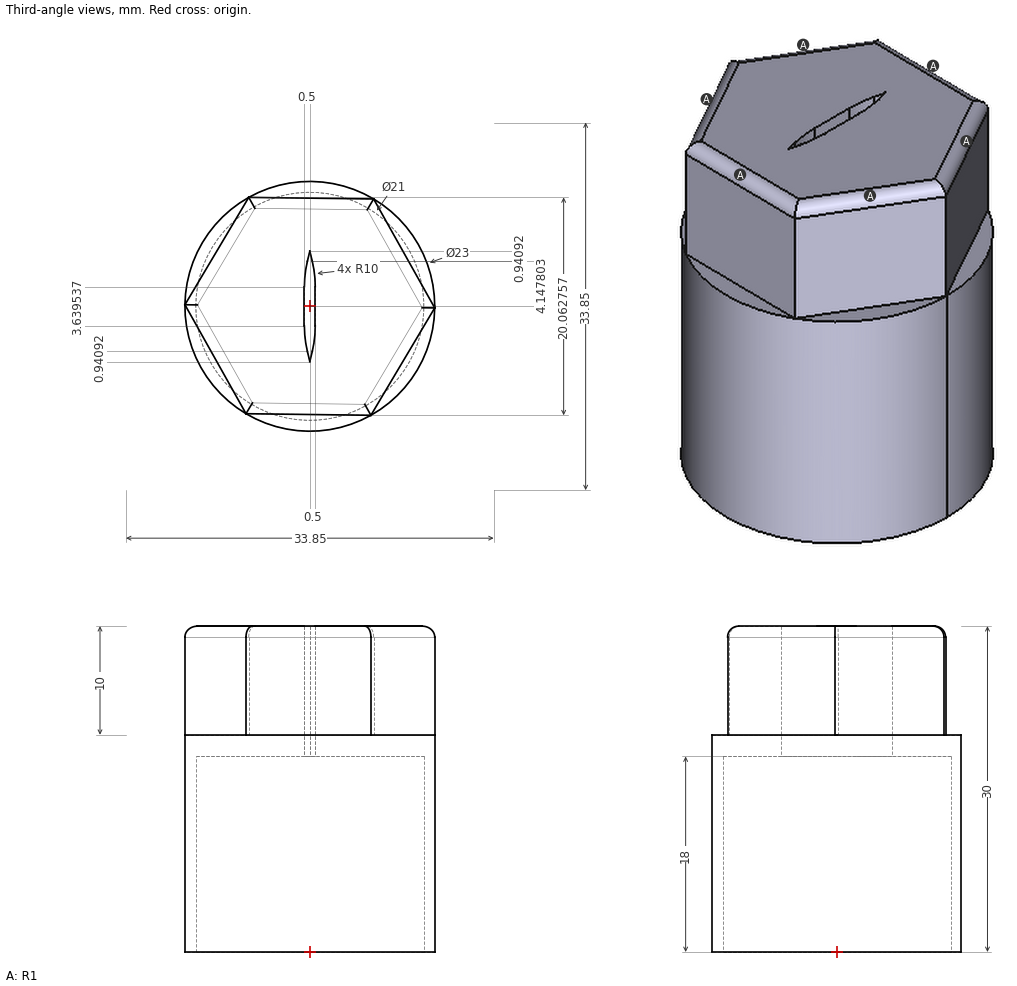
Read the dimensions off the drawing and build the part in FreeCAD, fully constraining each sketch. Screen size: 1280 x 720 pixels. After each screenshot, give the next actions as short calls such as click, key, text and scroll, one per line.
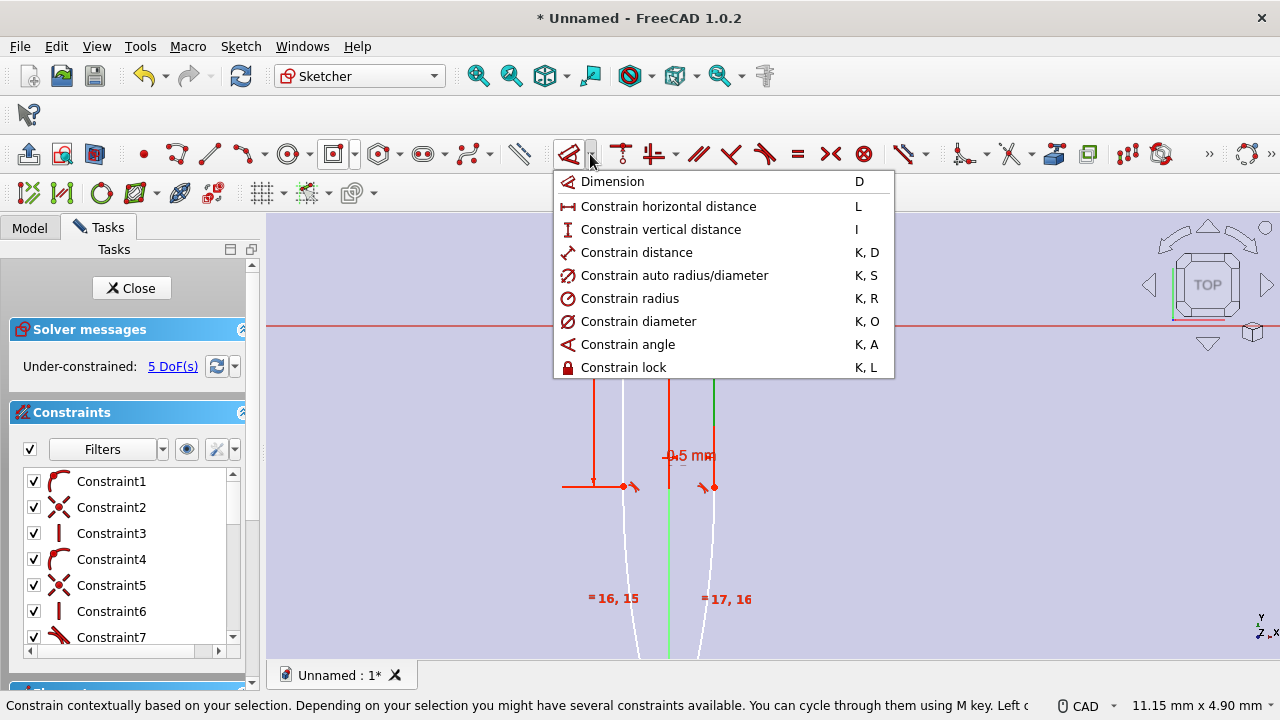
click(724, 230)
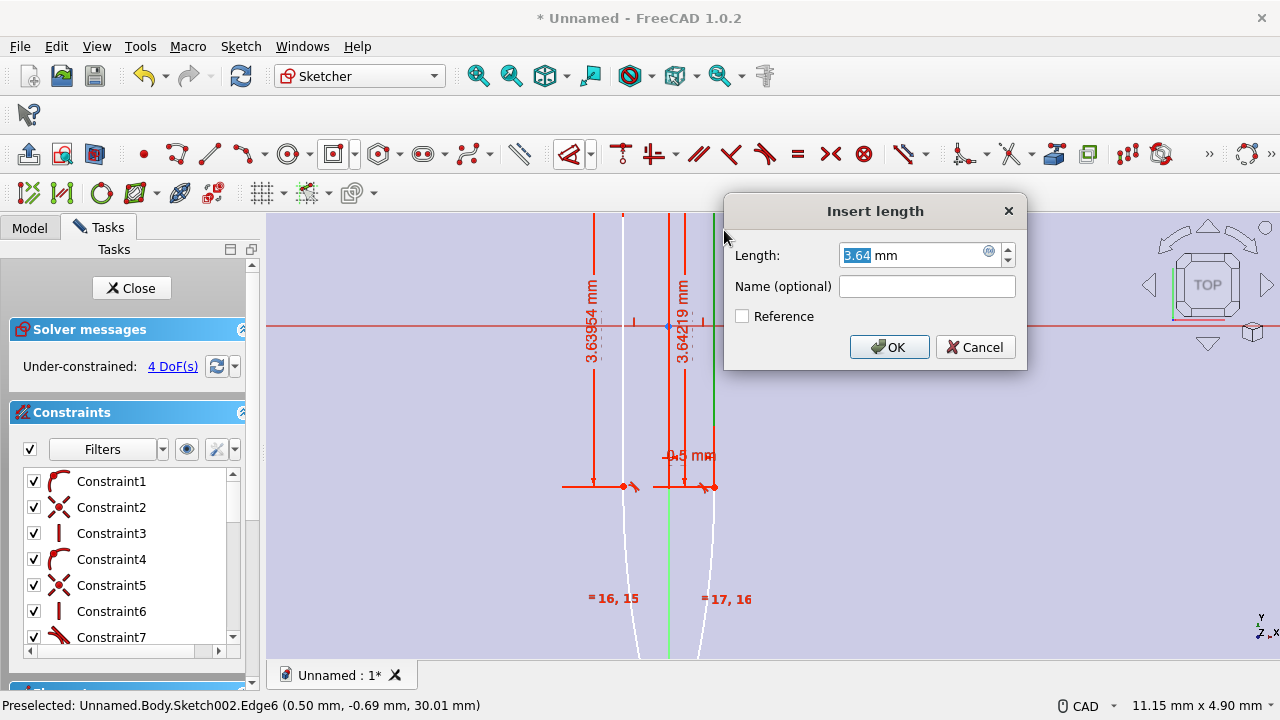
text(3.639537)
key(Return)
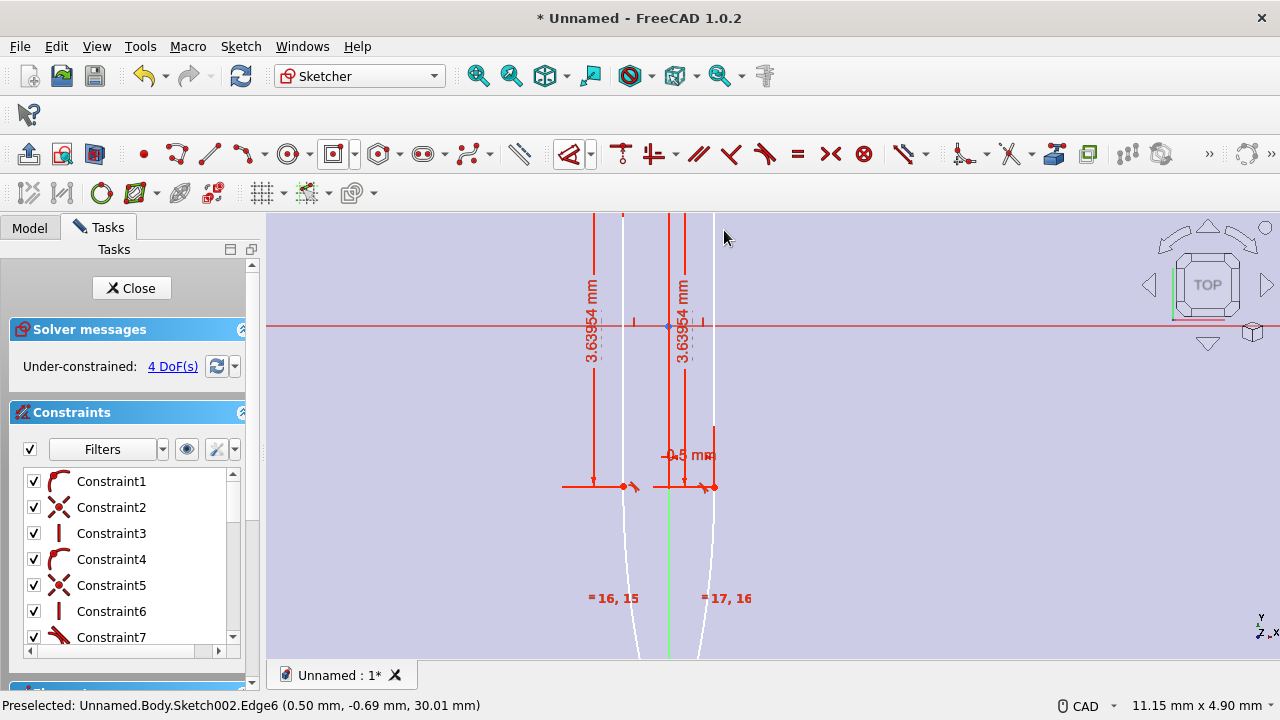
scroll(720, 483, down, 6)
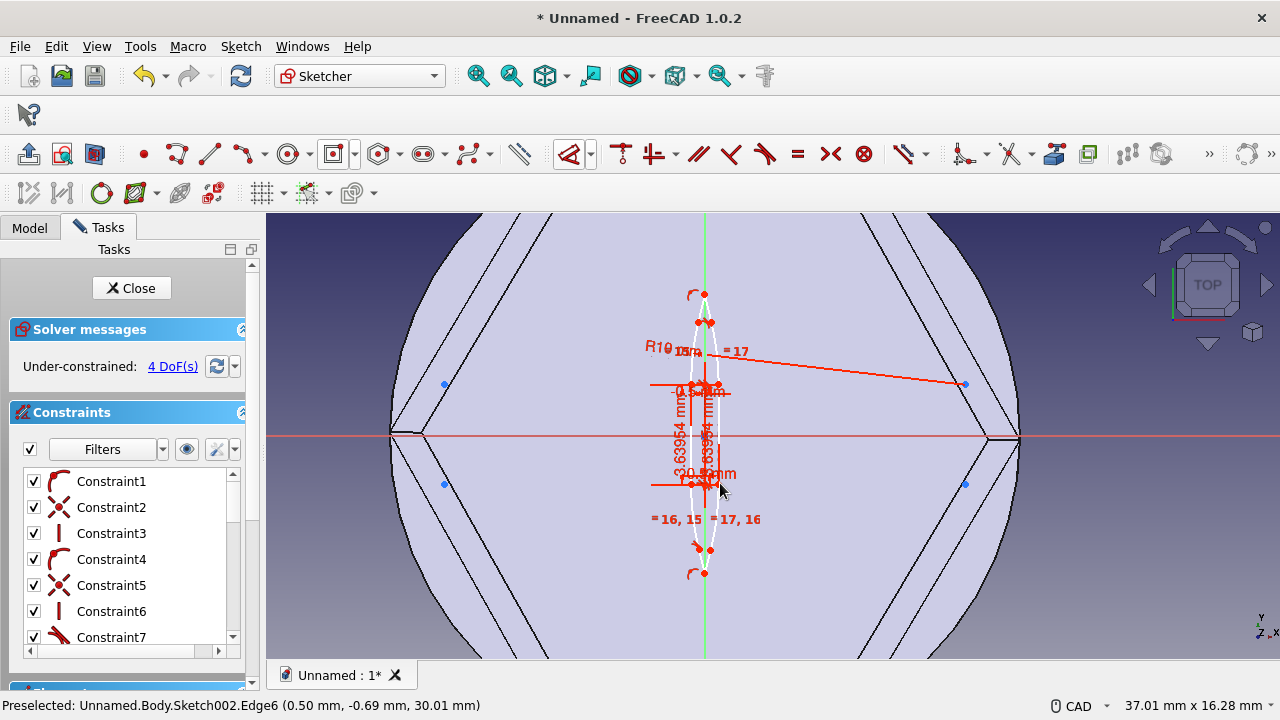
scroll(709, 314, up, 6)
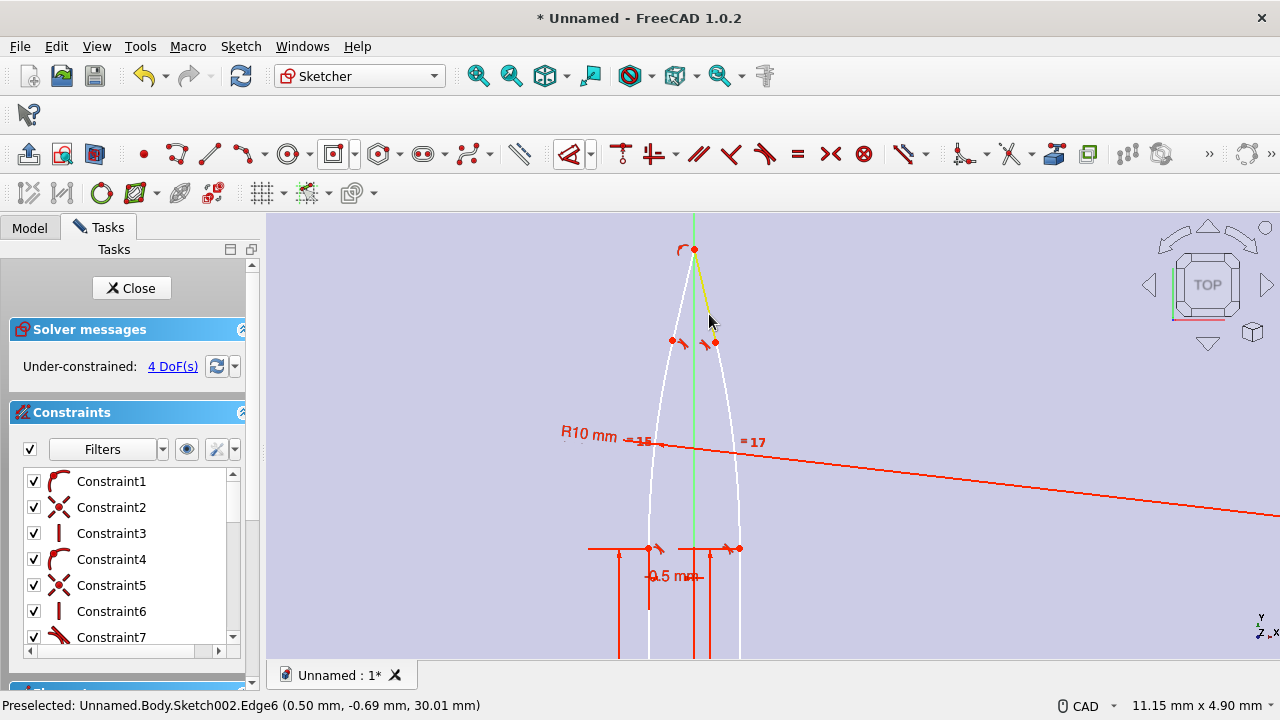
click(709, 314)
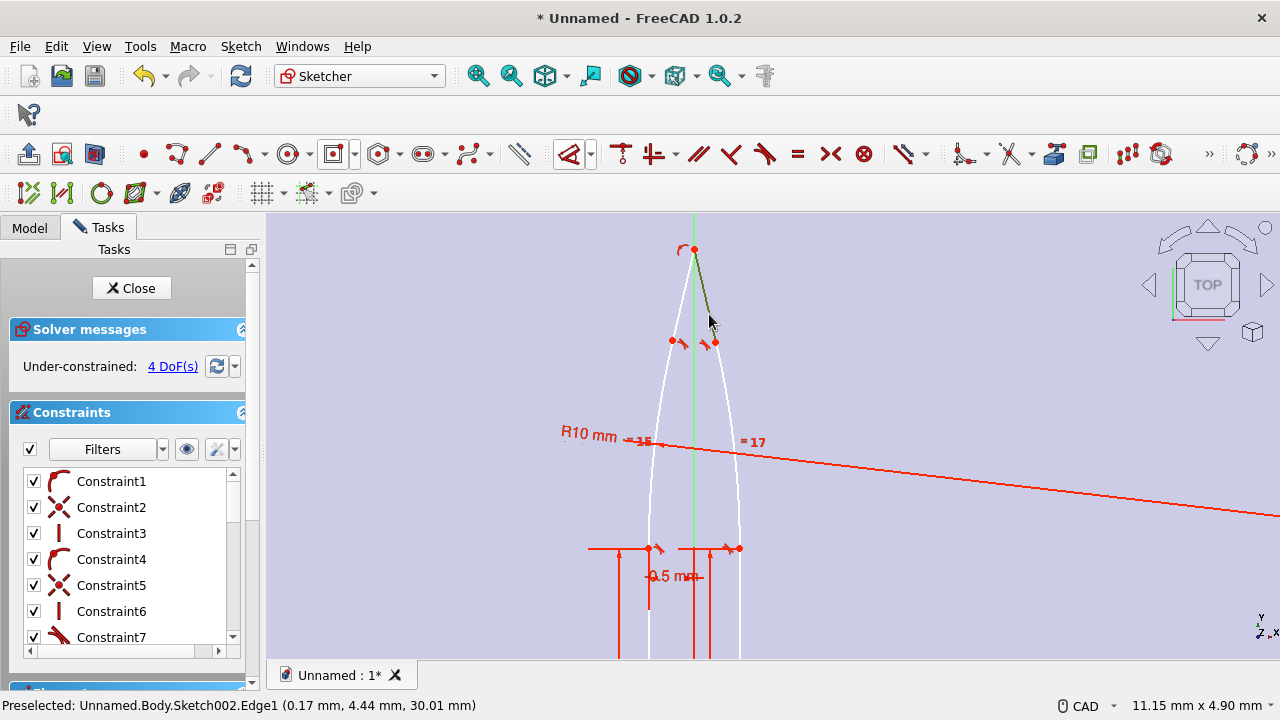
key(i)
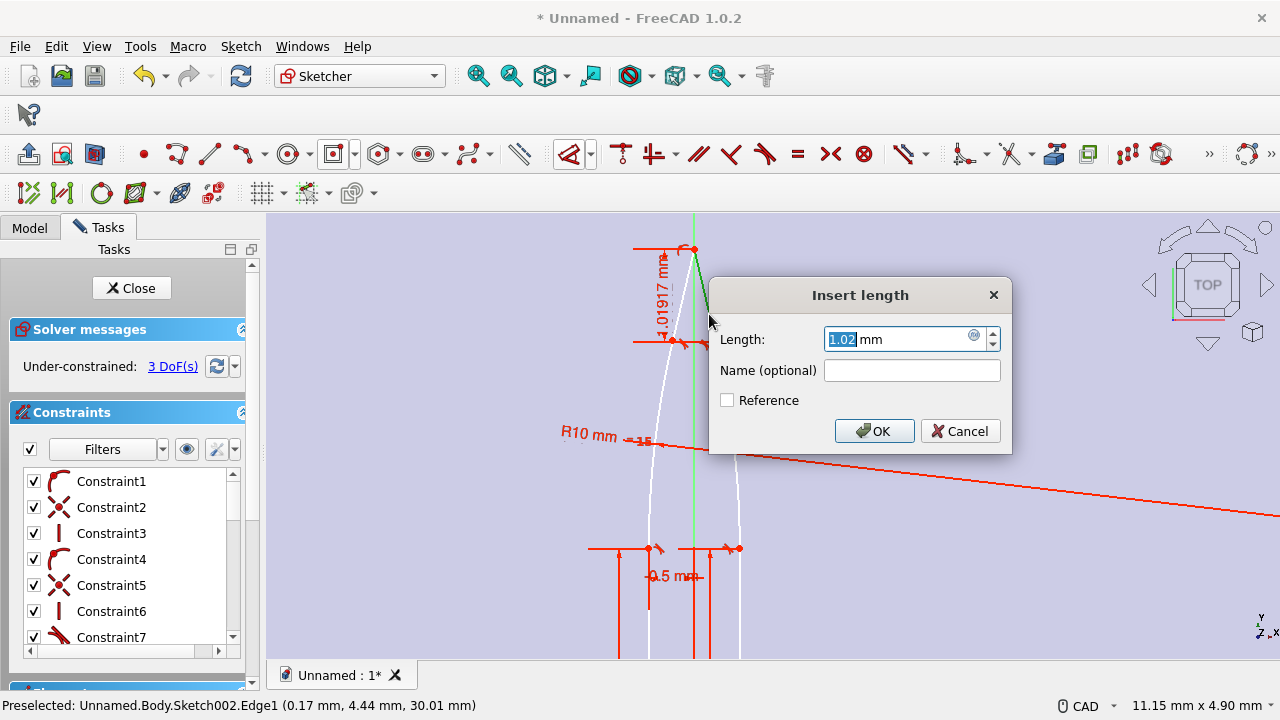
text(0.94092)
key(Return)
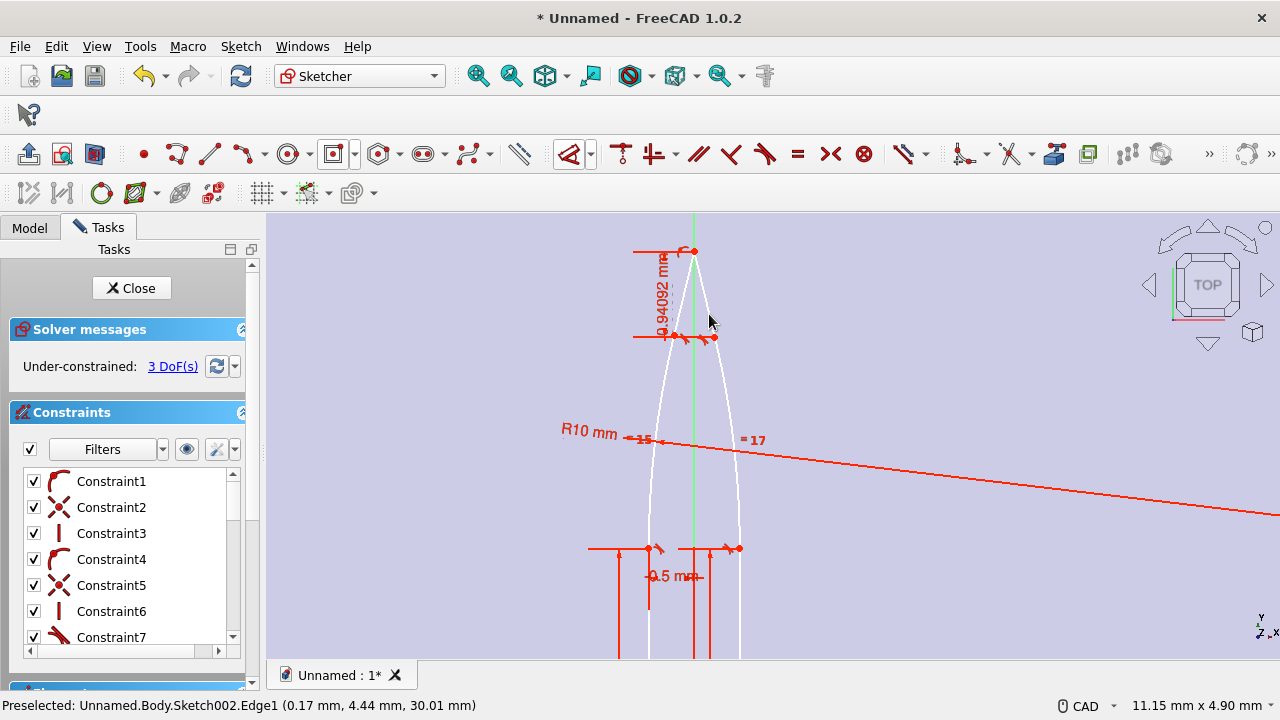
click(680, 311)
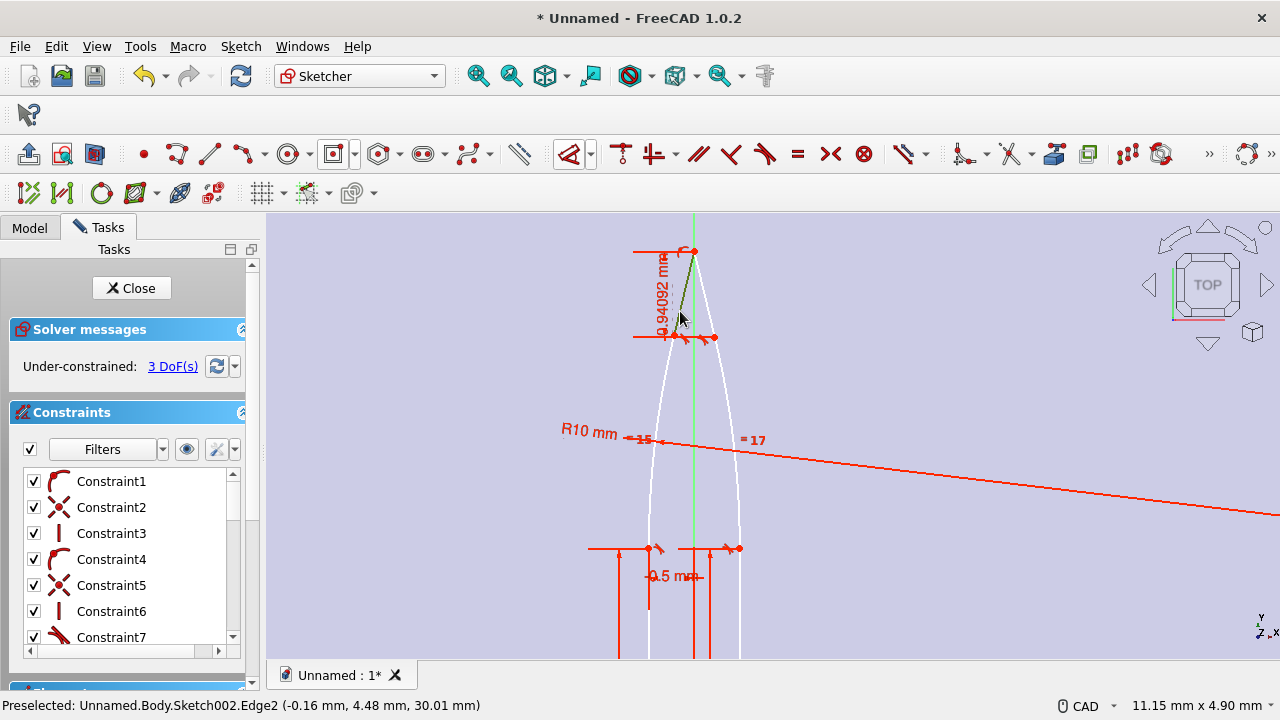
key(i)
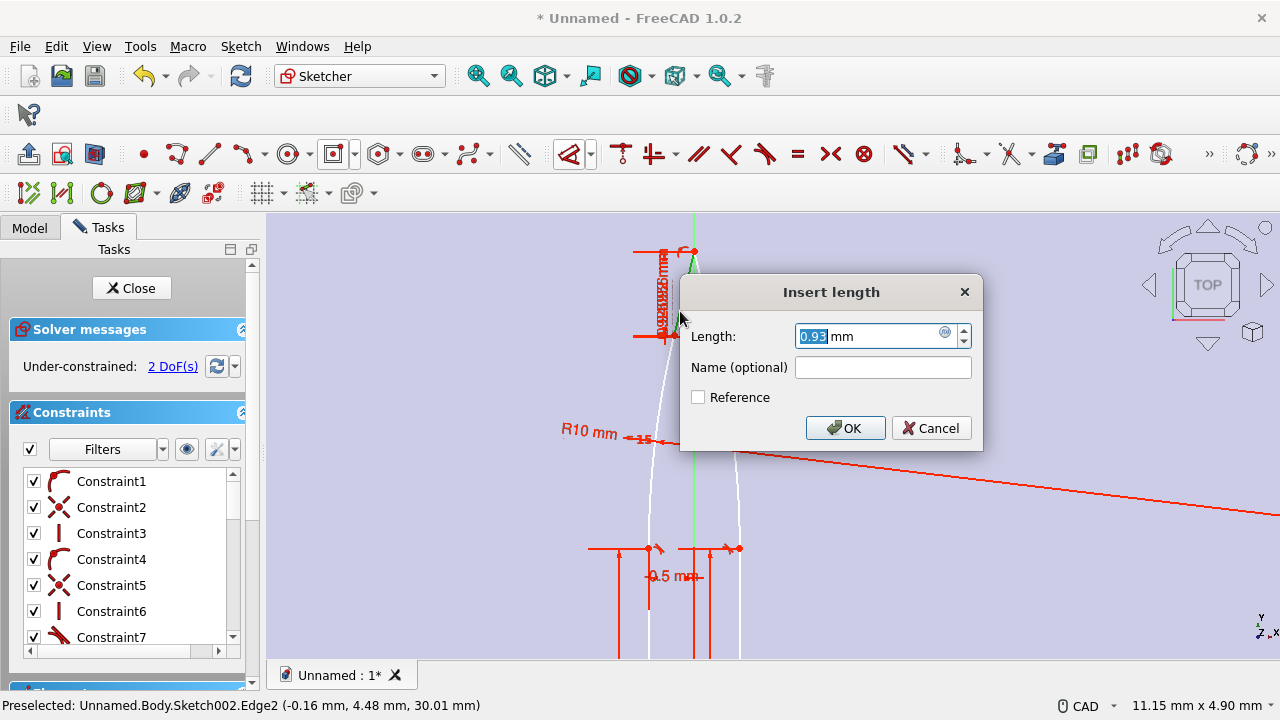
text(0.94092)
key(Return)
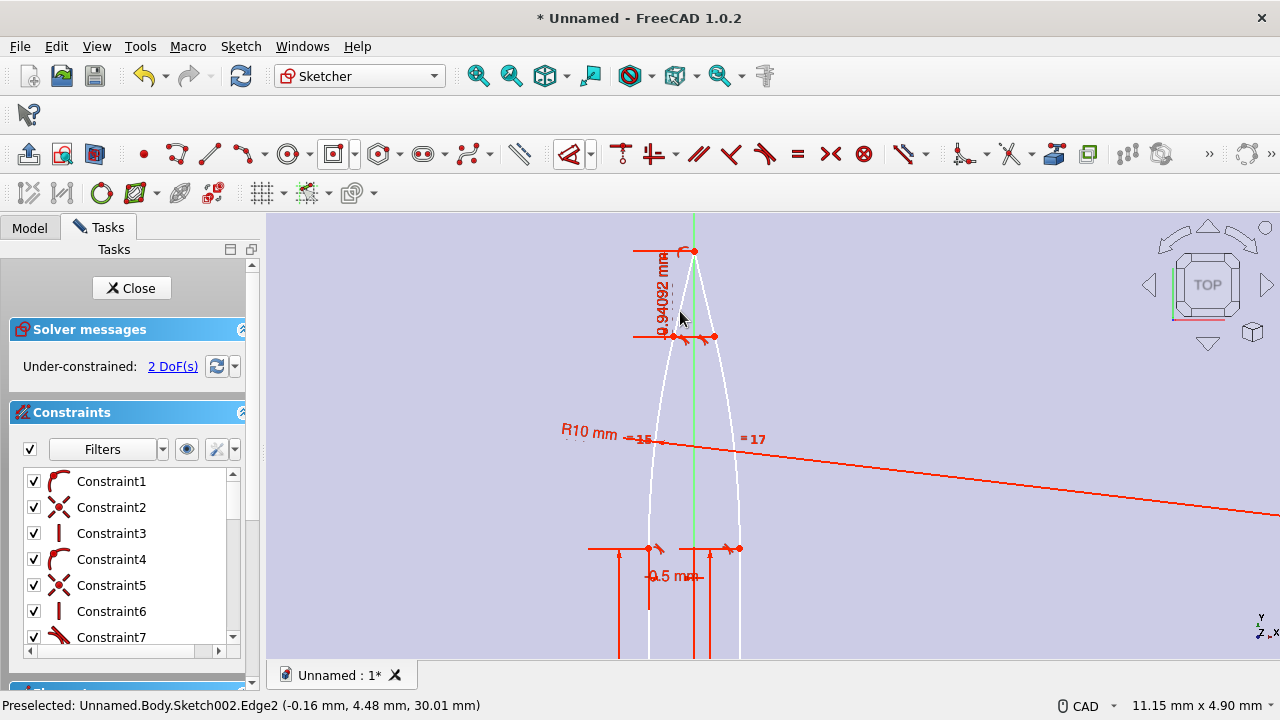
scroll(709, 314, down, 6)